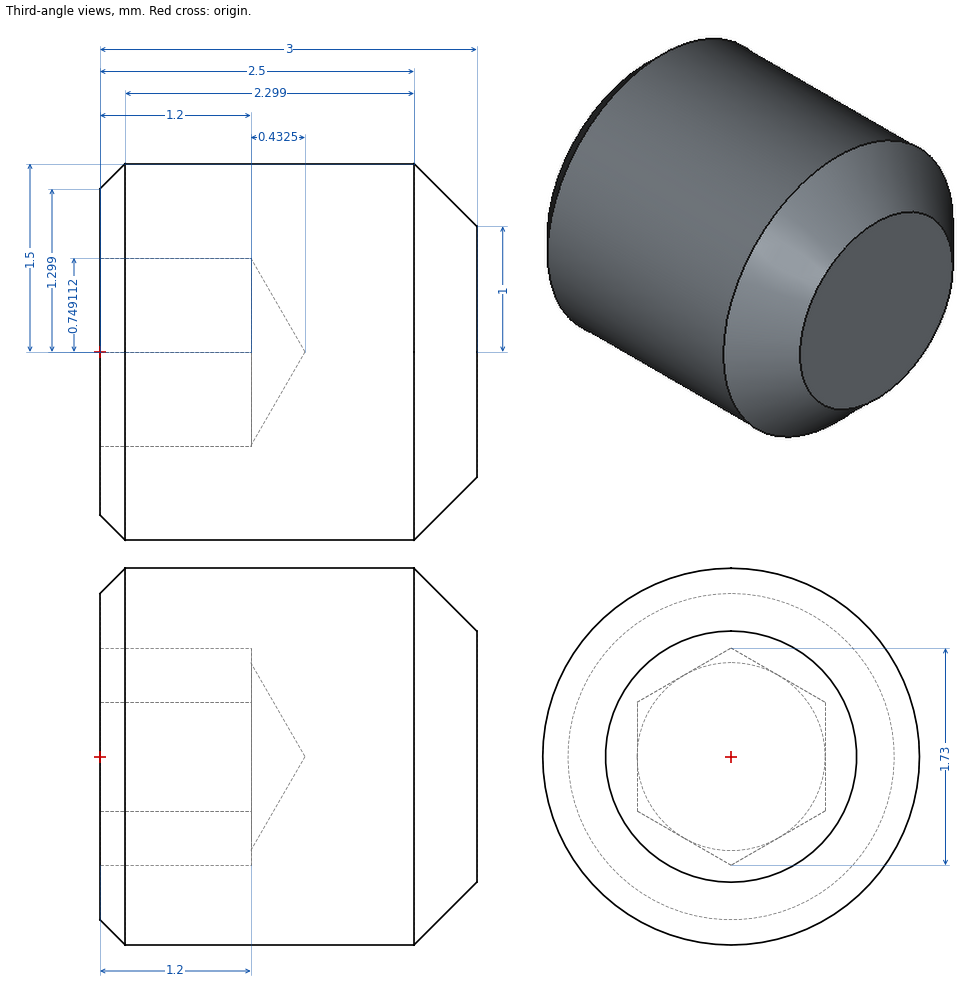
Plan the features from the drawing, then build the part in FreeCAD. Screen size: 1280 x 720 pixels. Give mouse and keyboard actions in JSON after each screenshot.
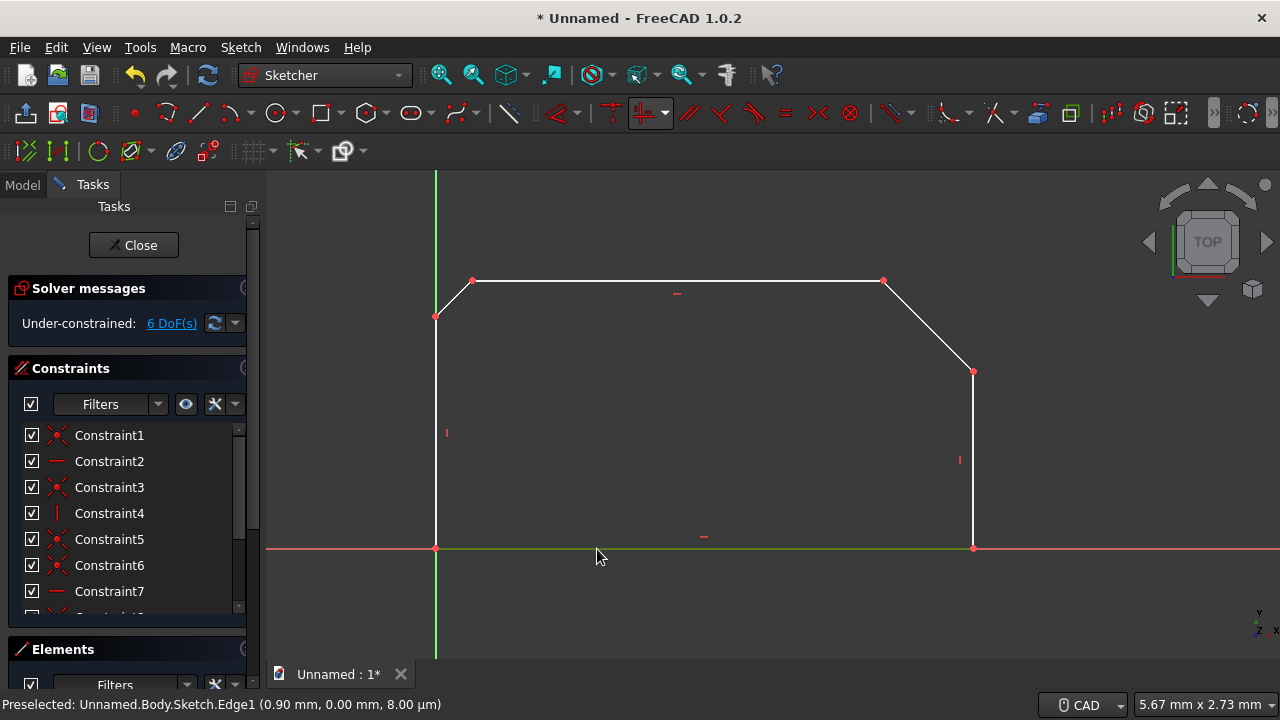
{"action": "key", "text": "l"}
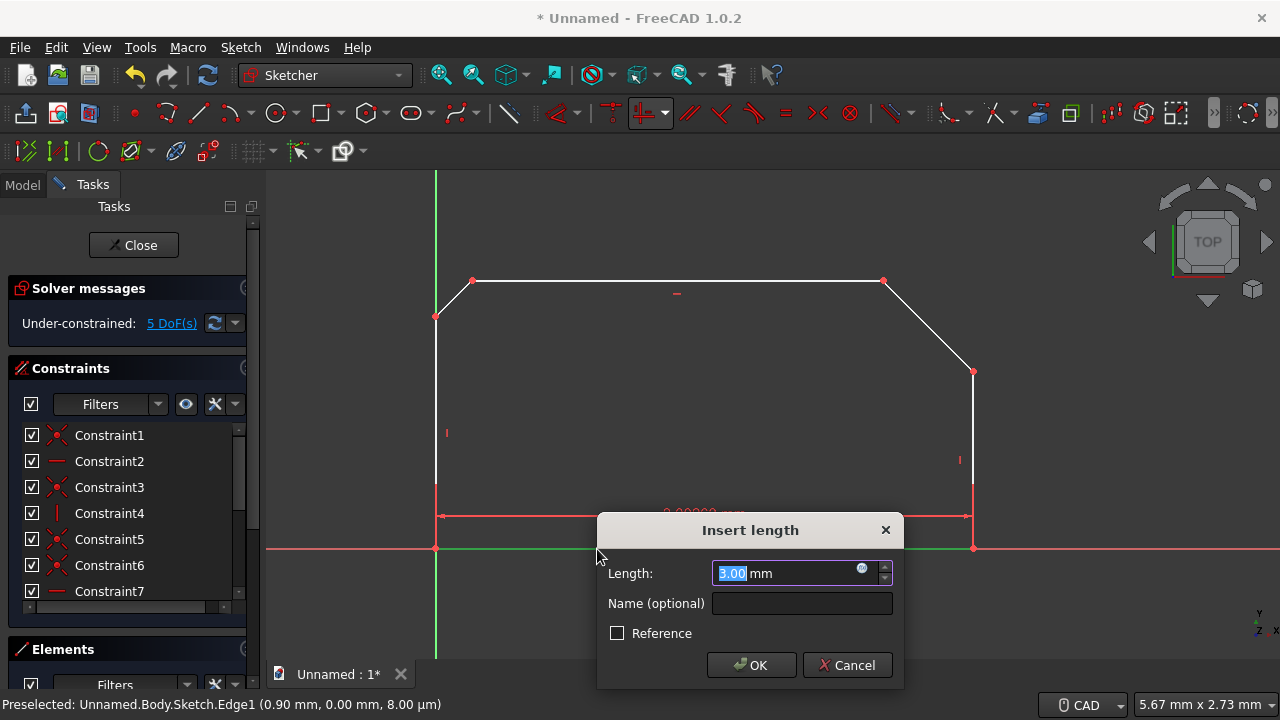
{"action": "type", "text": "3"}
{"action": "key", "text": "Return"}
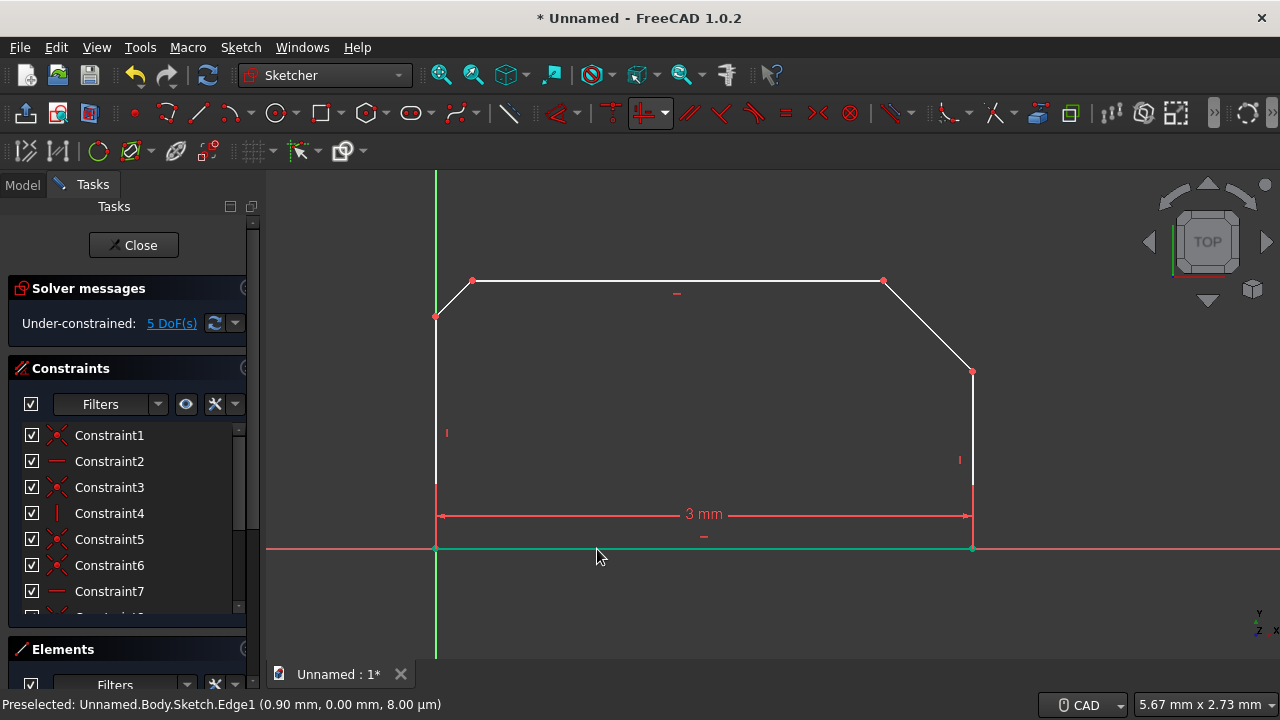
{"action": "left_click", "coordinate": [973, 495]}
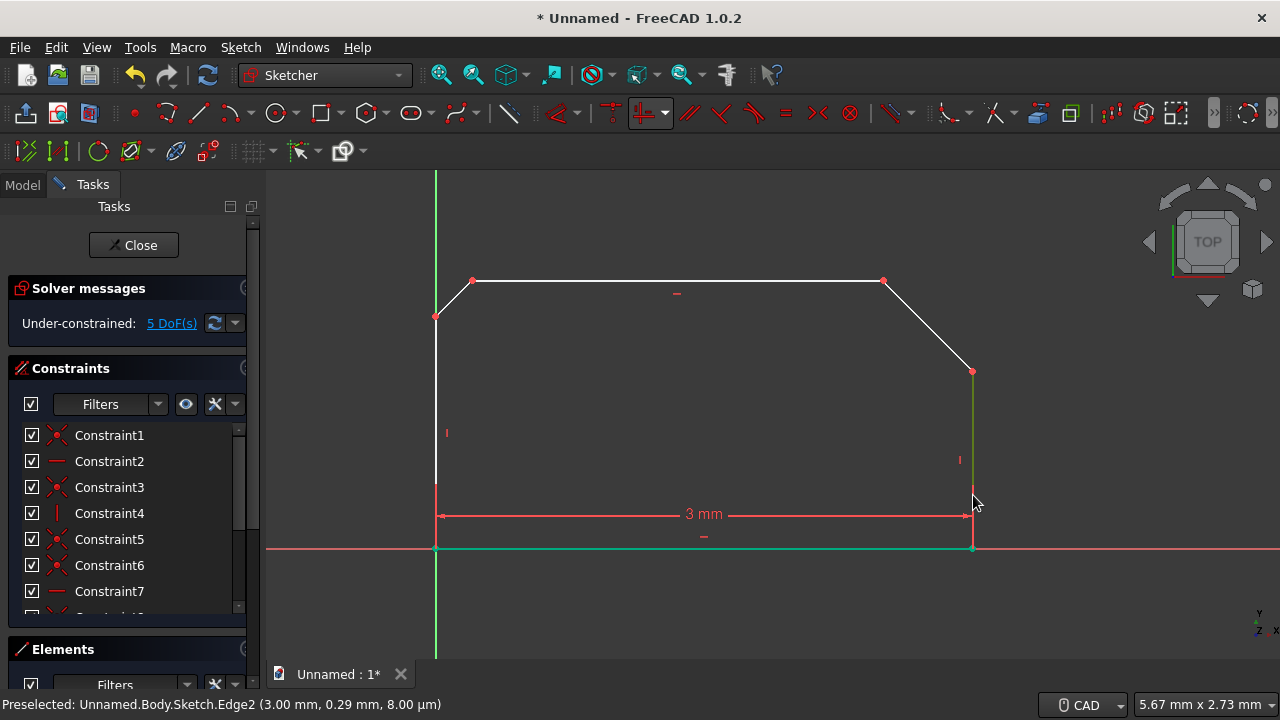
{"action": "left_click", "coordinate": [580, 114]}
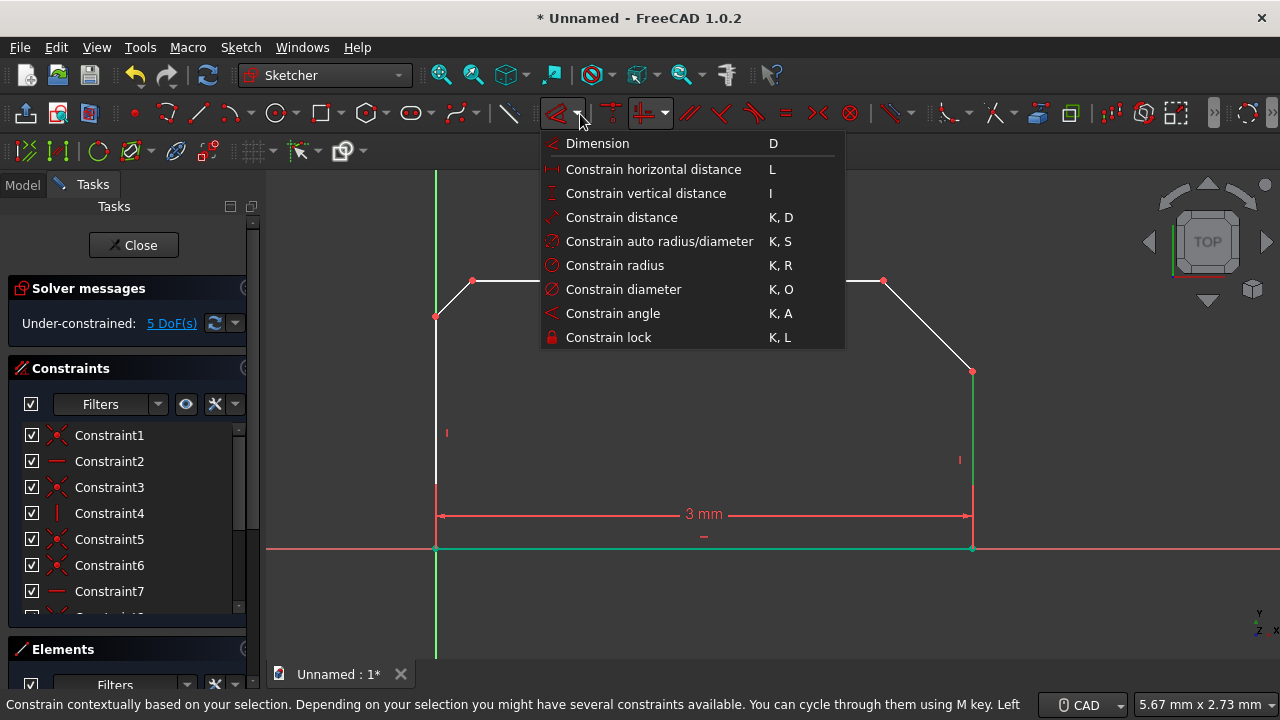
{"action": "left_click", "coordinate": [693, 193]}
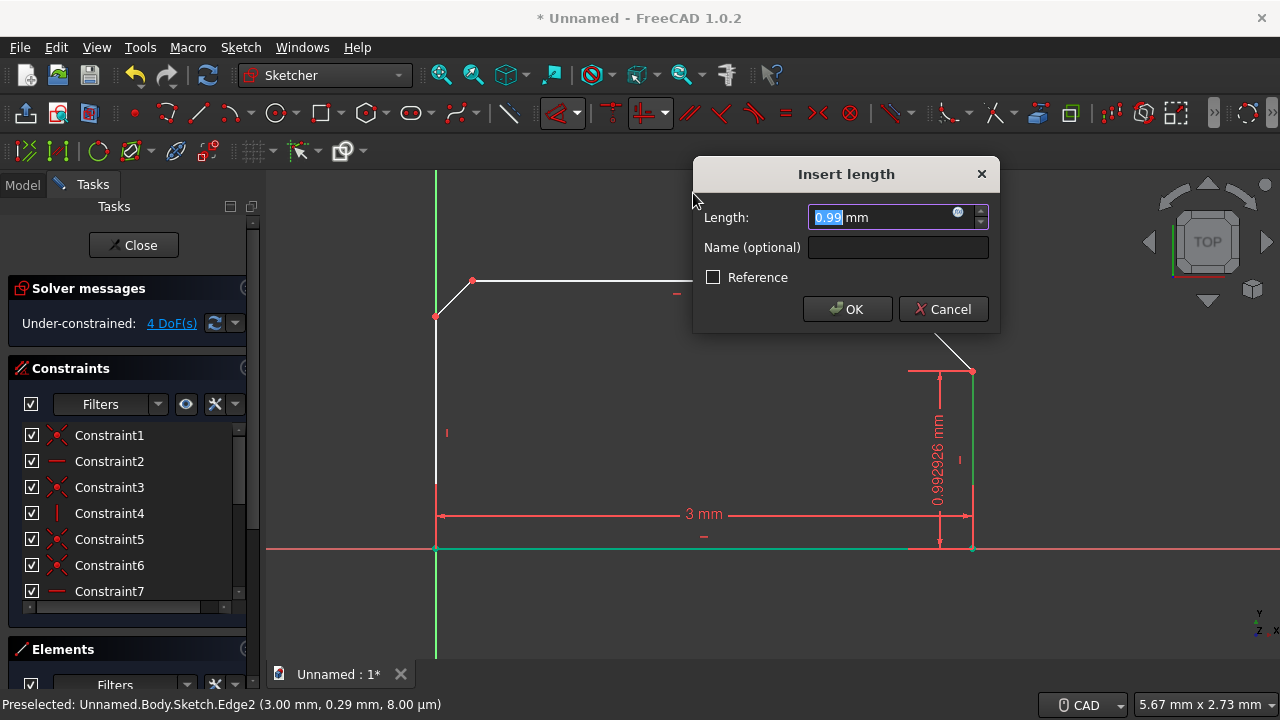
{"action": "type", "text": "1"}
{"action": "key", "text": "Return"}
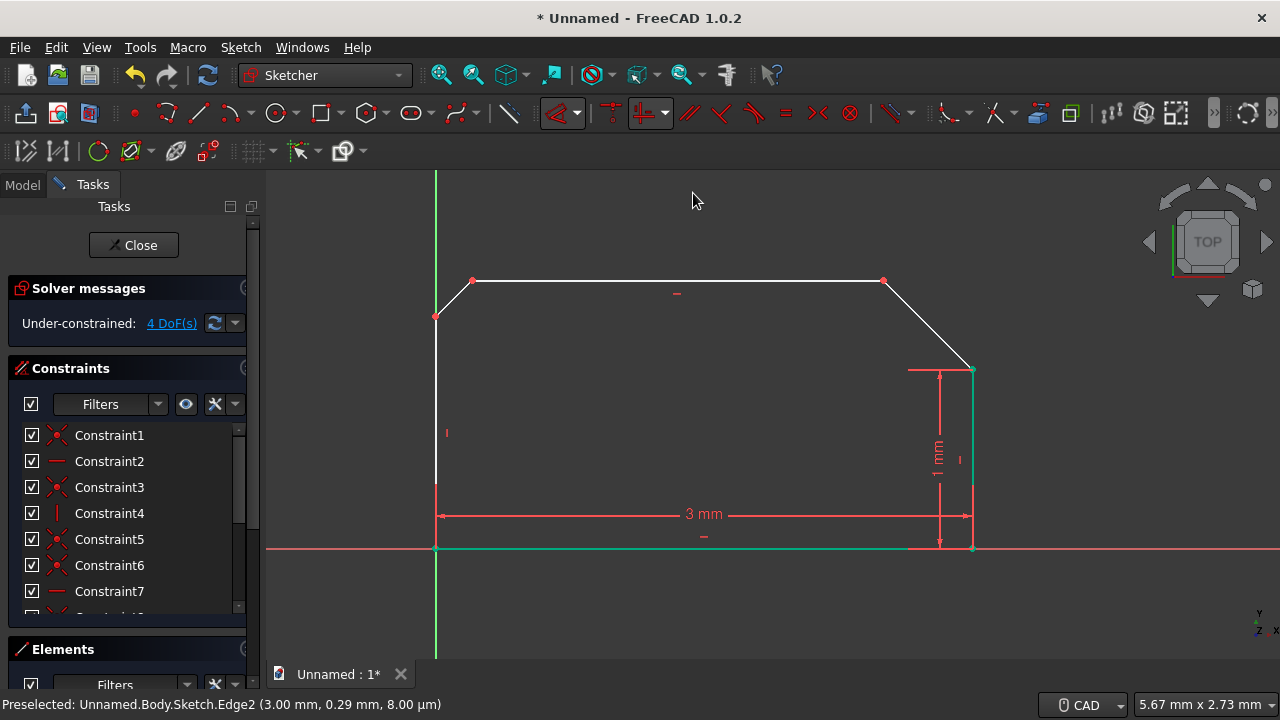
{"action": "left_click", "coordinate": [883, 281]}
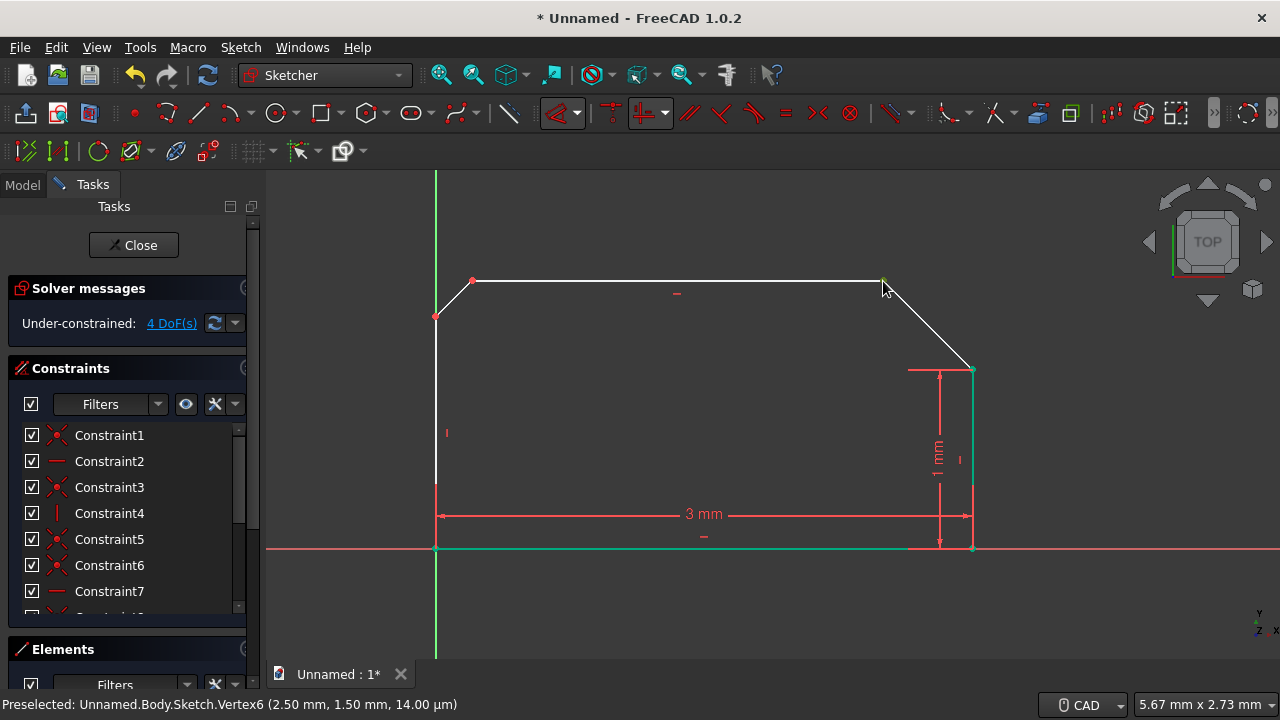
{"action": "key", "text": "l"}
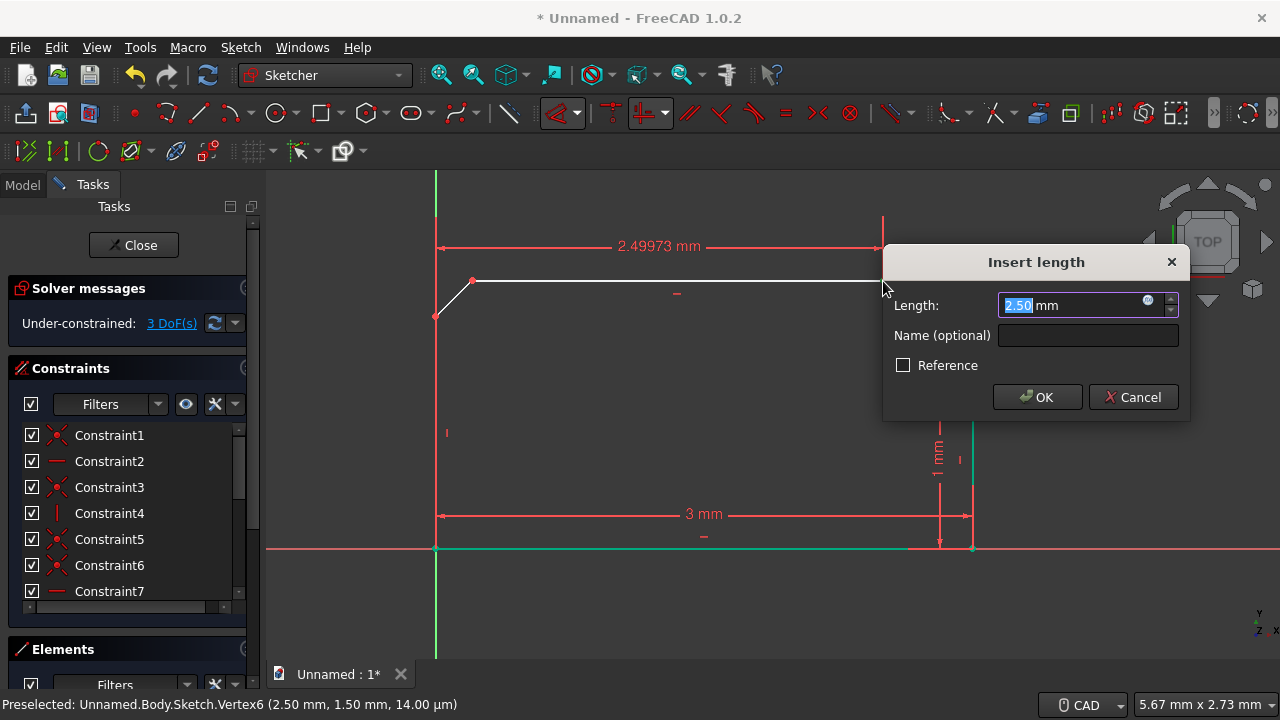
{"action": "type", "text": "2.5"}
{"action": "key", "text": "Return"}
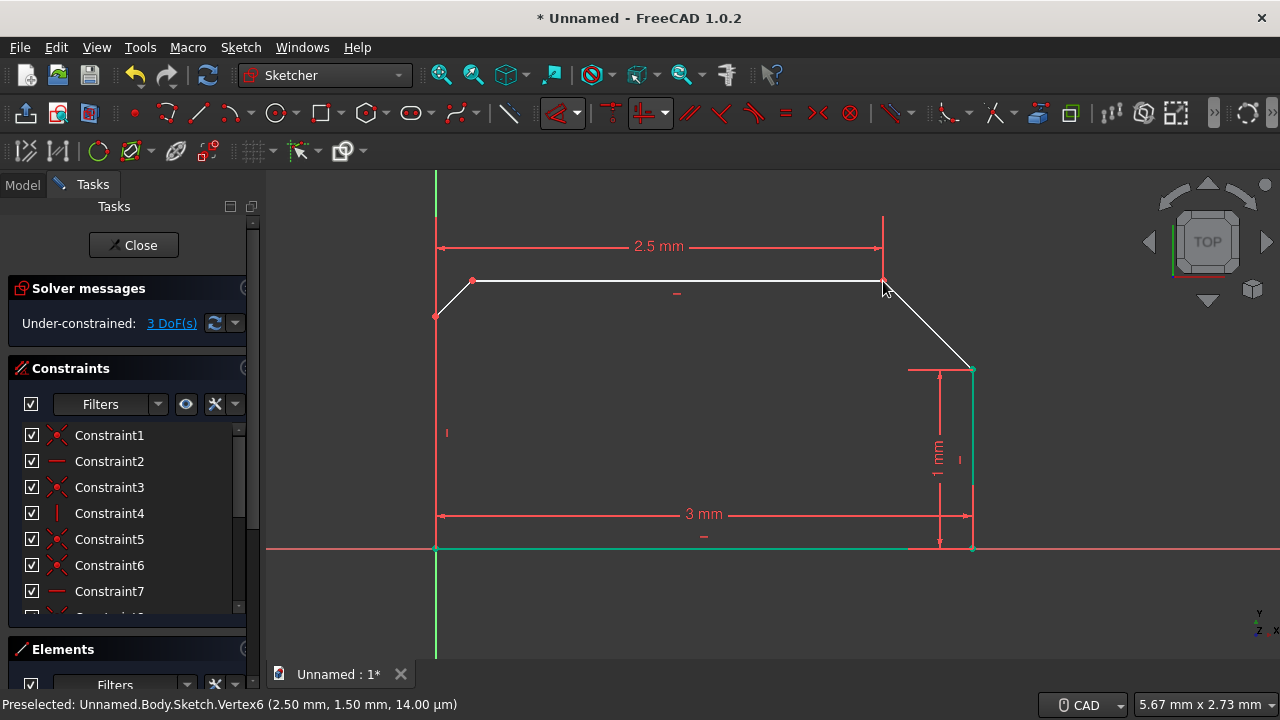
{"action": "left_click", "coordinate": [883, 281]}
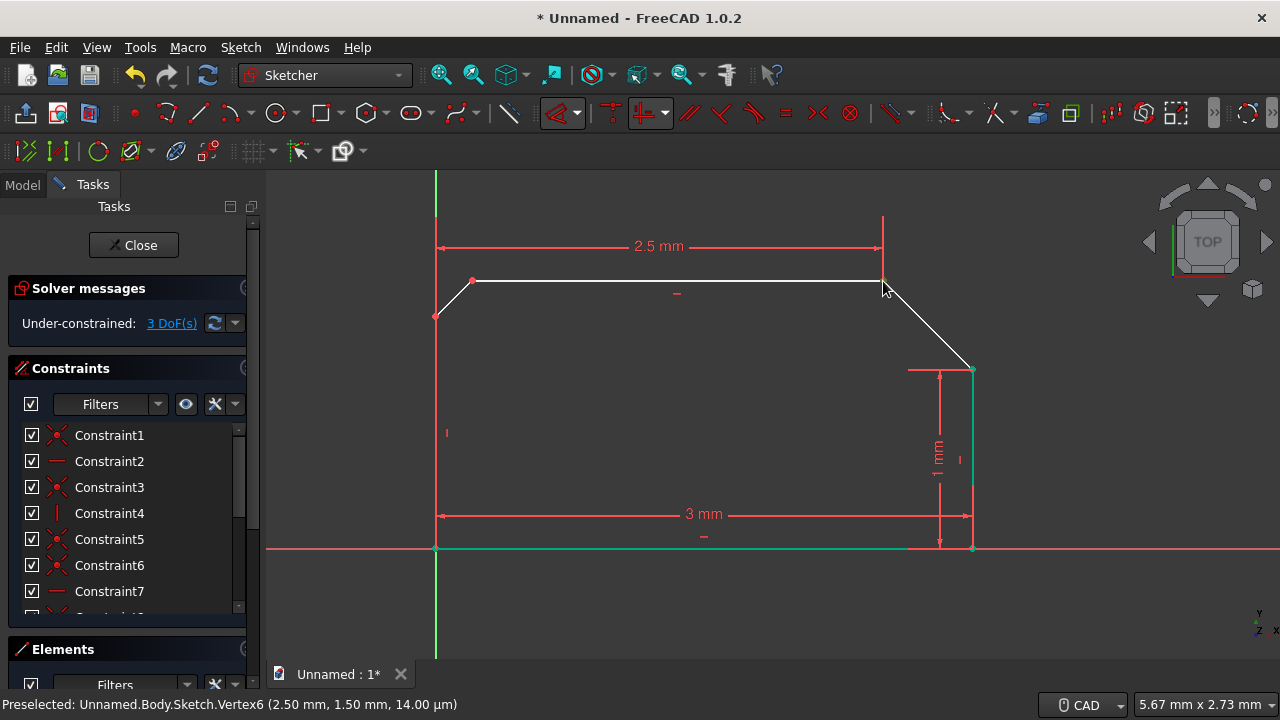
{"action": "left_click", "coordinate": [580, 114]}